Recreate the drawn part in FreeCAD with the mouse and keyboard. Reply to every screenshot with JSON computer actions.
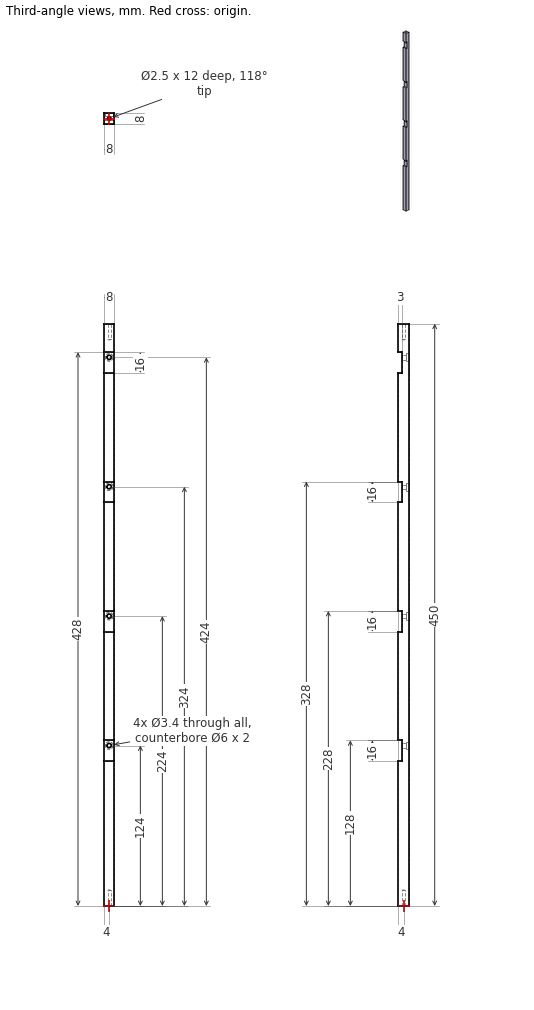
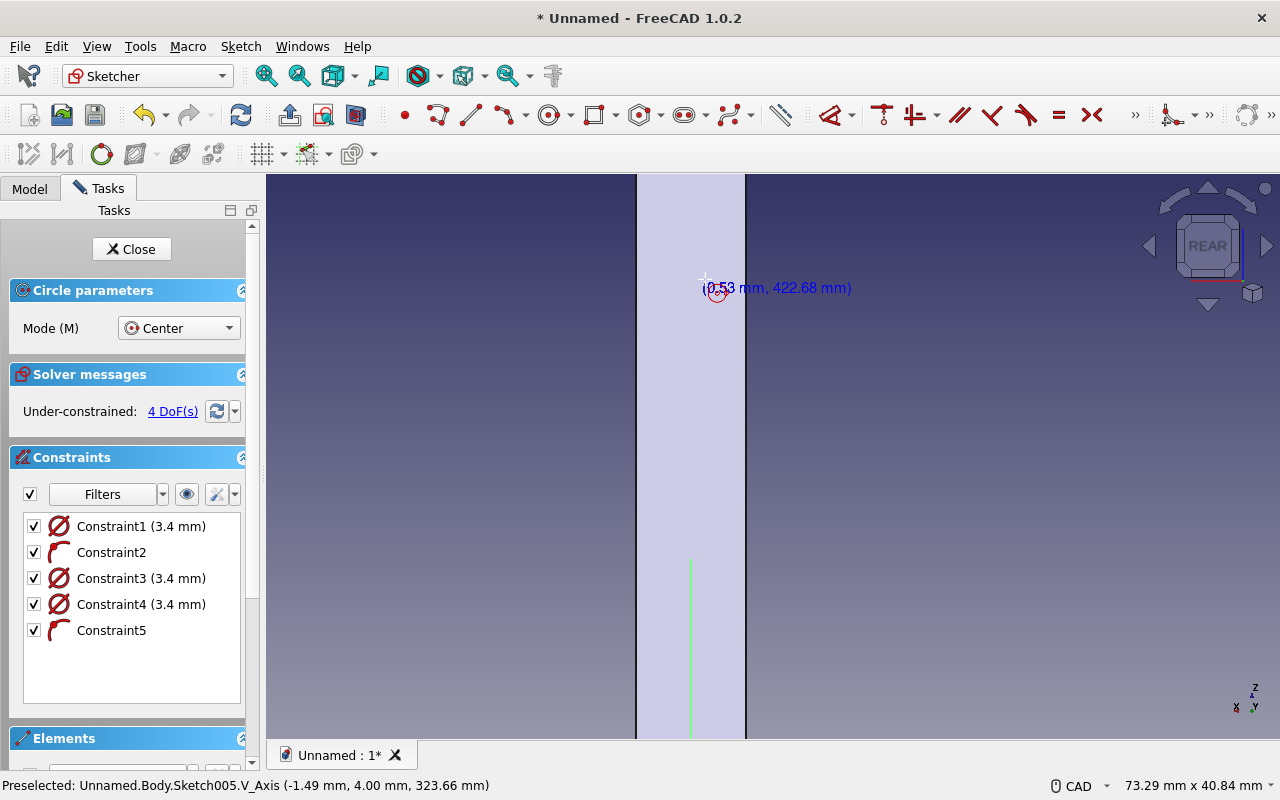
{"action": "scroll", "coordinate": [705, 279], "scroll_direction": "down", "scroll_amount": 14}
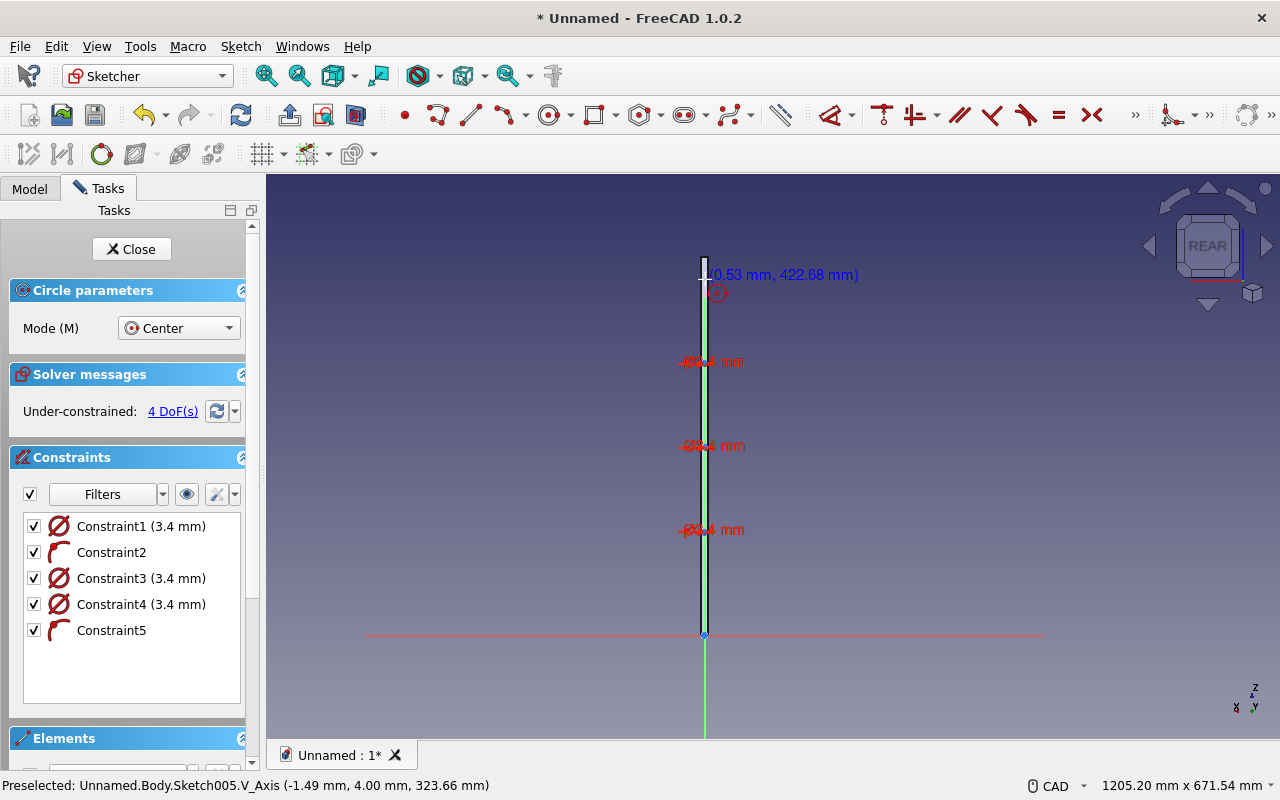
{"action": "left_click", "coordinate": [705, 279]}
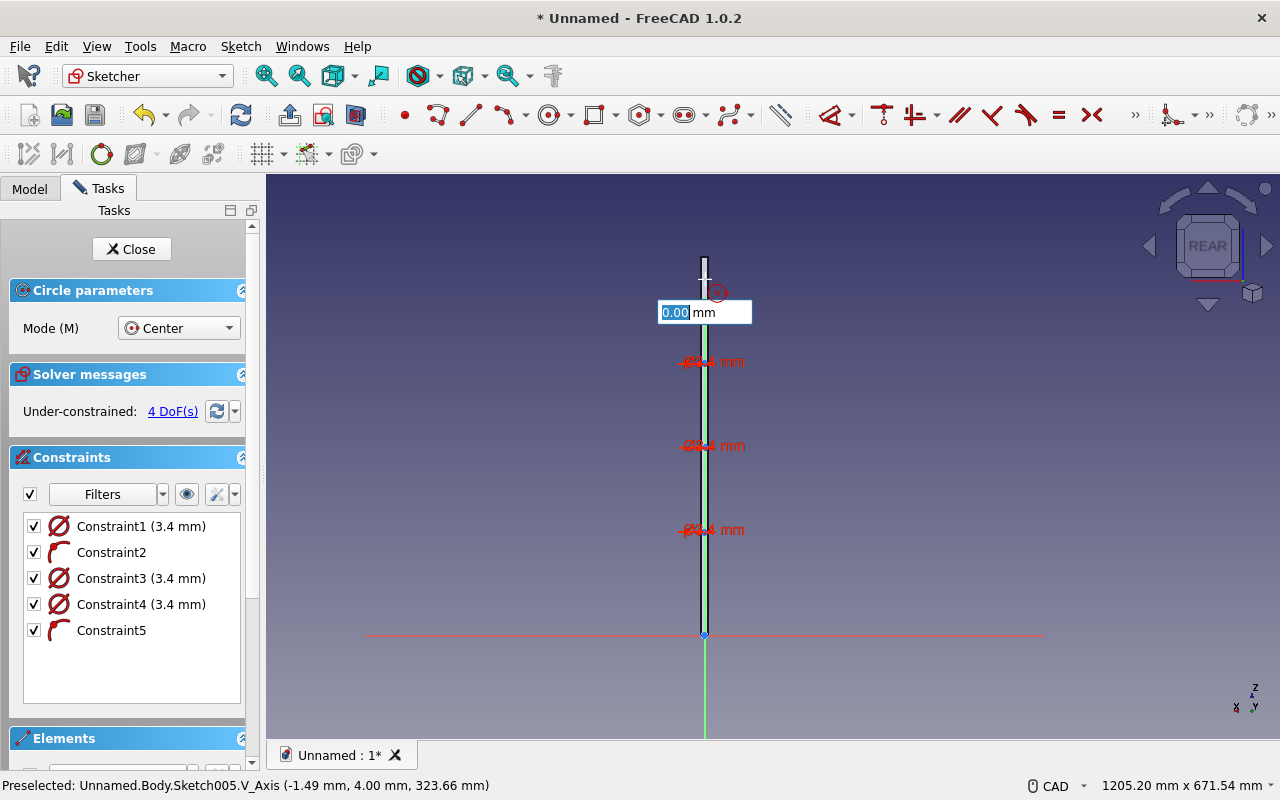
{"action": "scroll", "coordinate": [706, 278], "scroll_direction": "up", "scroll_amount": 13}
{"action": "mouse_move", "coordinate": [699, 281]}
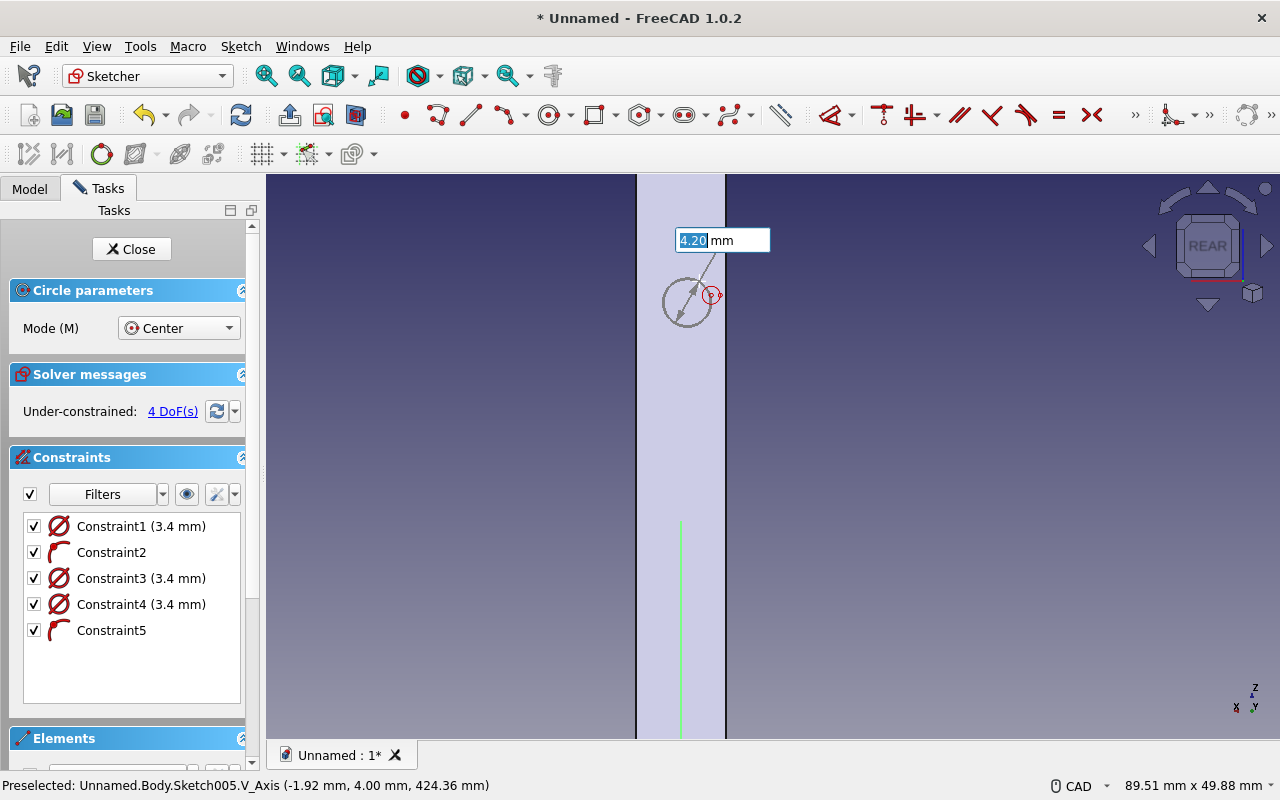
{"action": "type", "text": "3.4"}
{"action": "key", "text": "Return"}
{"action": "key", "text": "Escape"}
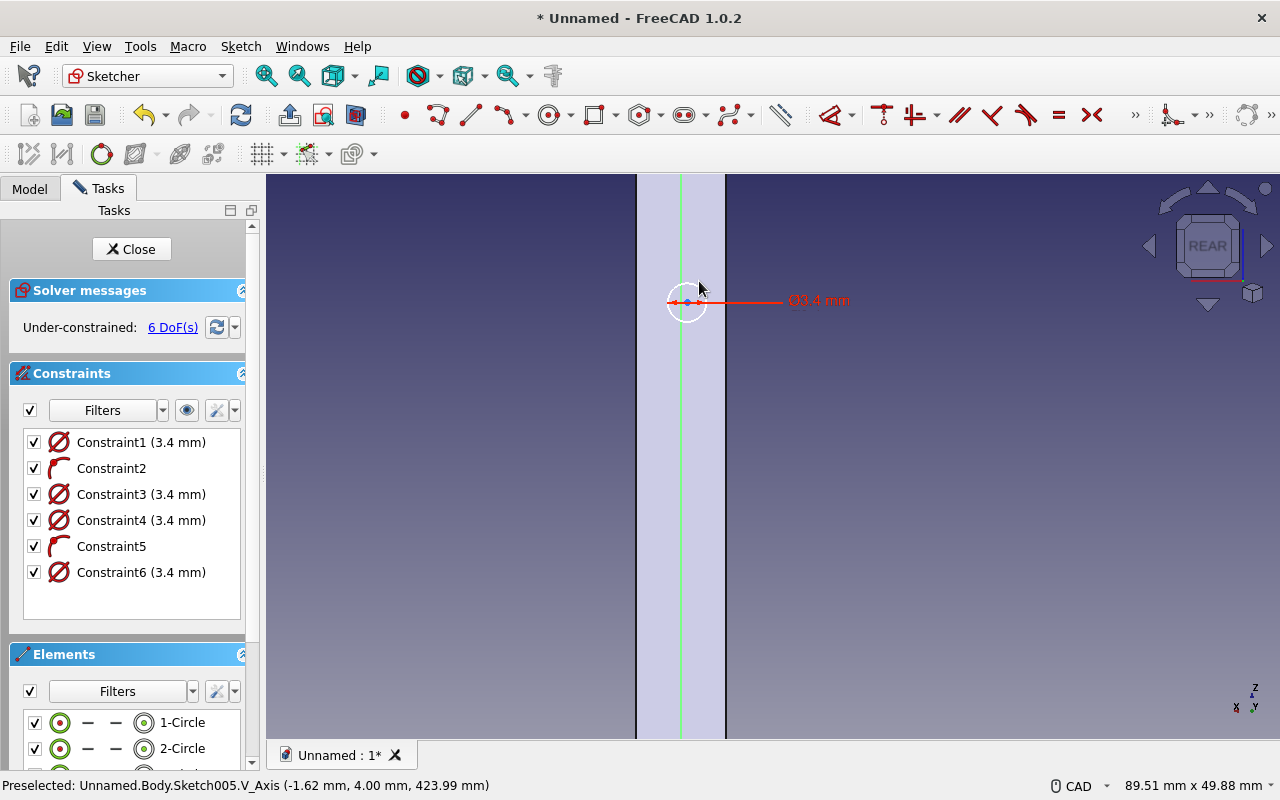
{"action": "scroll", "coordinate": [706, 278], "scroll_direction": "down", "scroll_amount": 13}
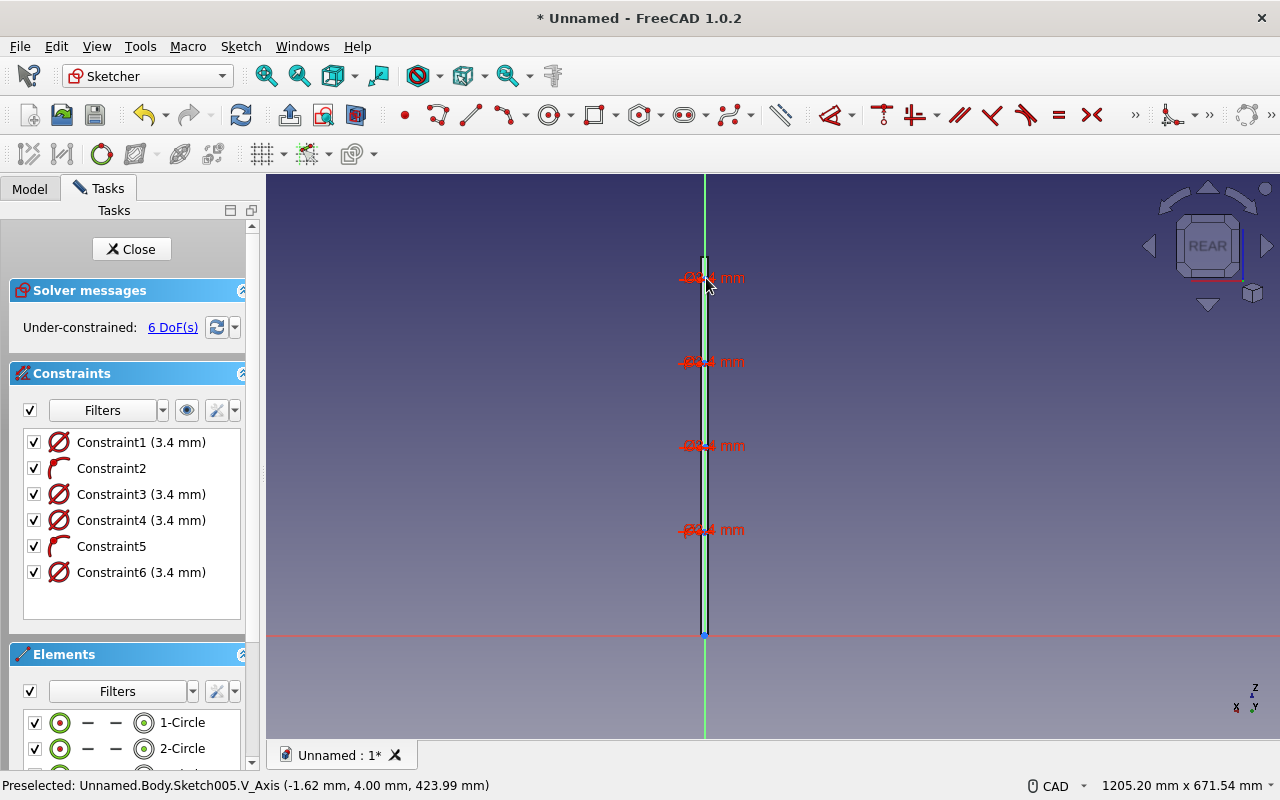
{"action": "left_click", "coordinate": [705, 448]}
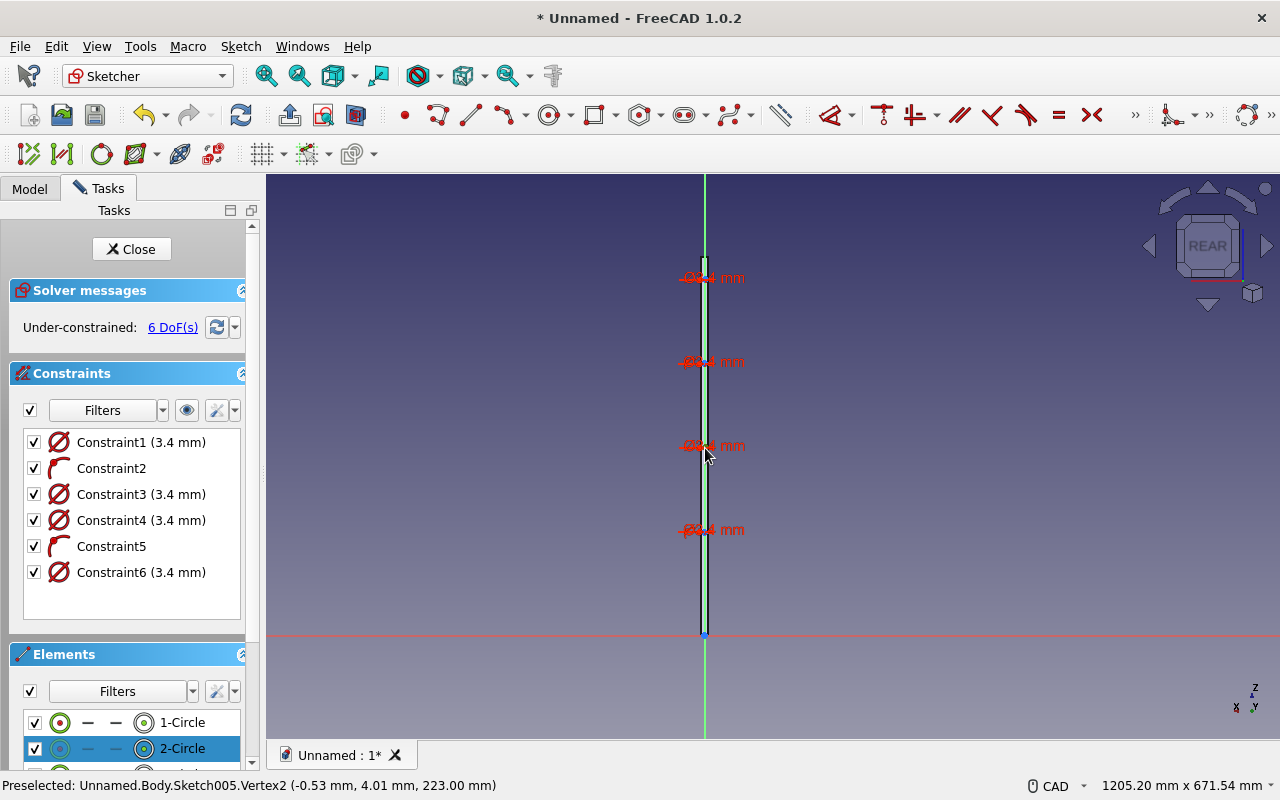
{"action": "left_click", "coordinate": [705, 675]}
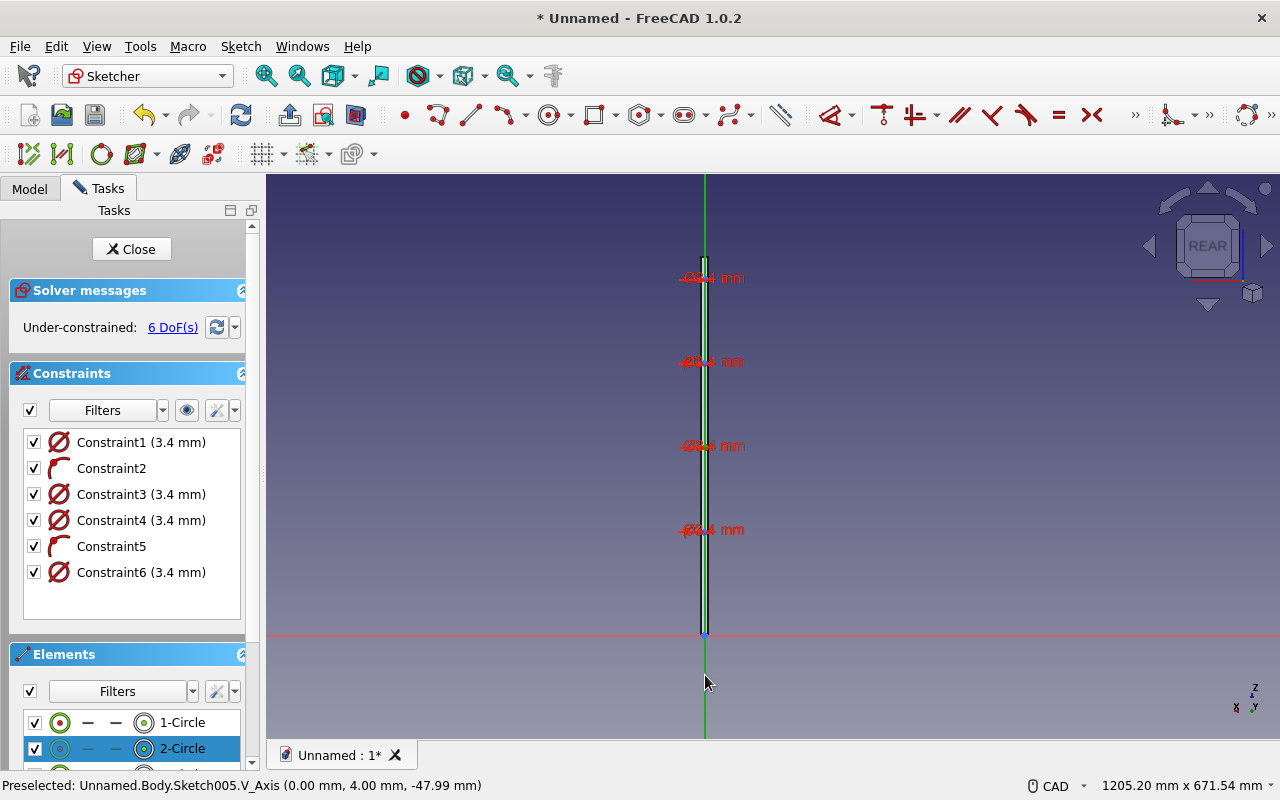
{"action": "key", "text": "c"}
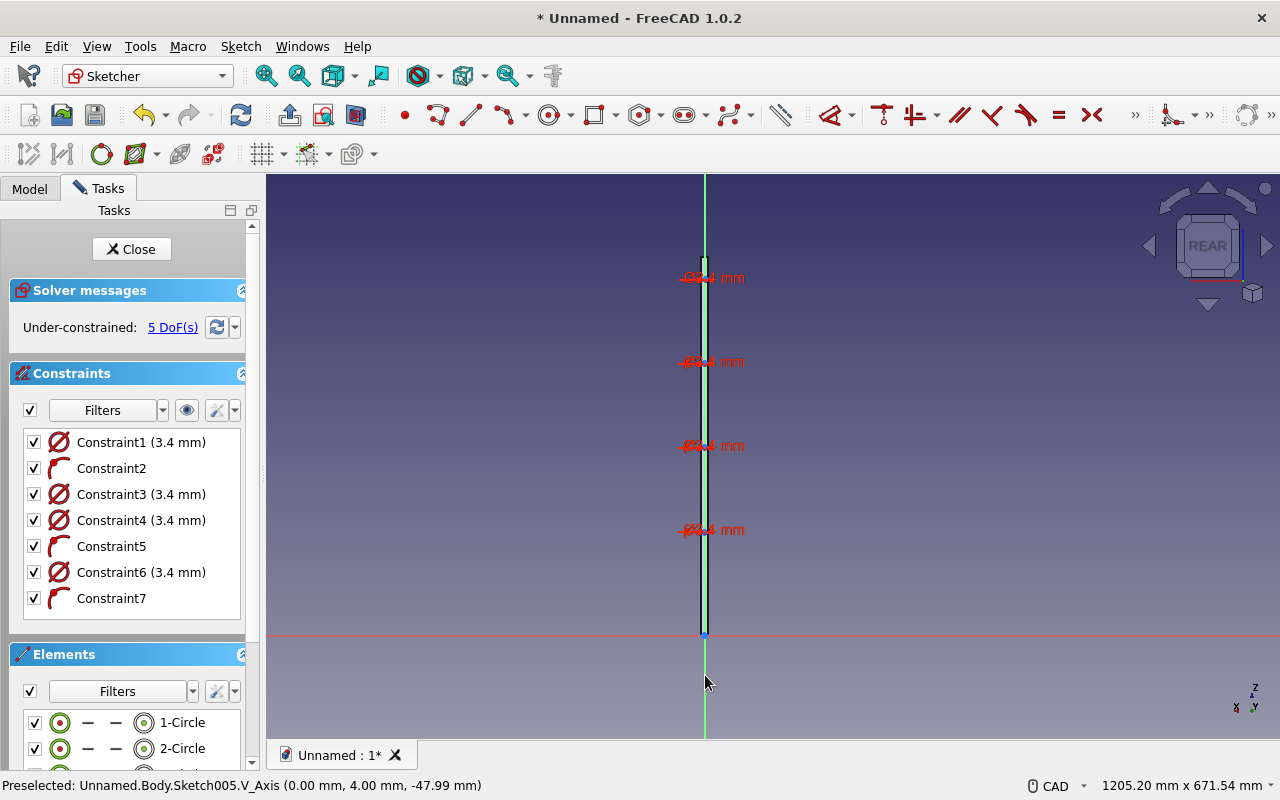
{"action": "left_click", "coordinate": [705, 280]}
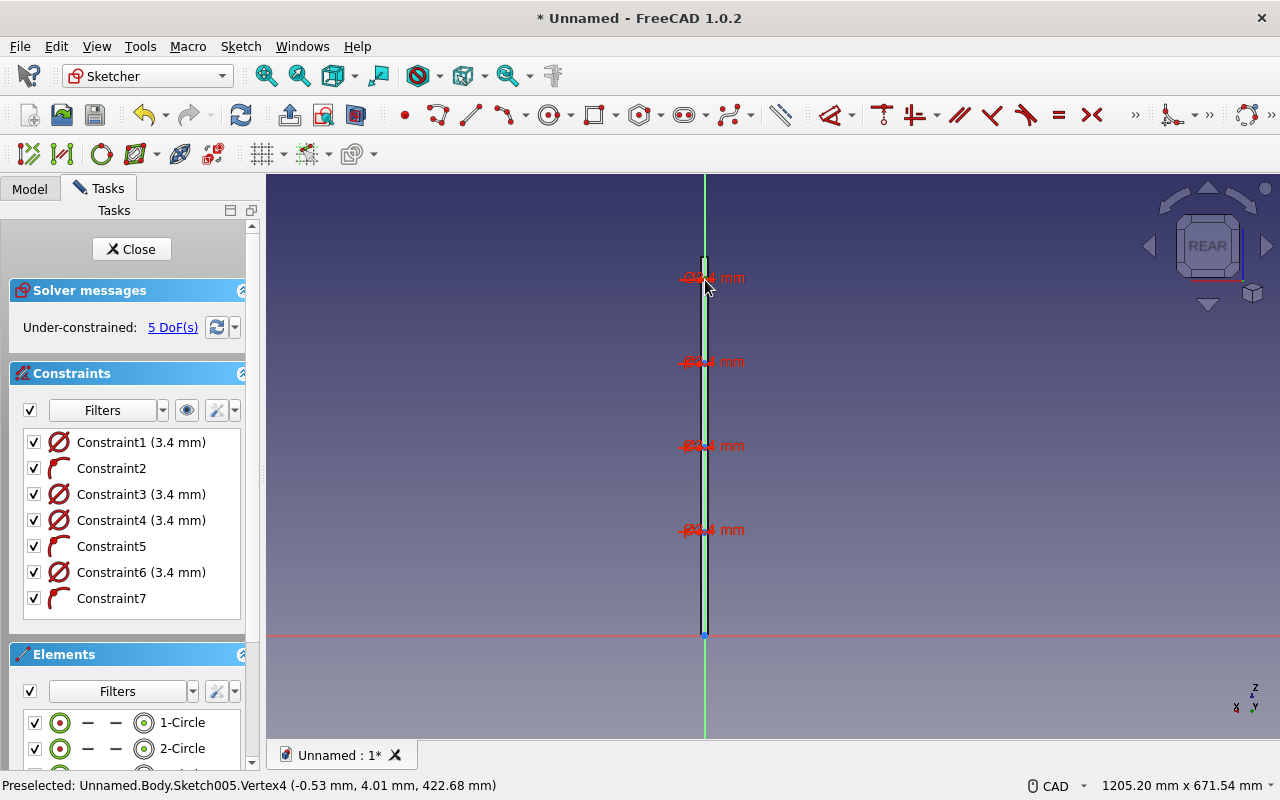
{"action": "left_click", "coordinate": [705, 675]}